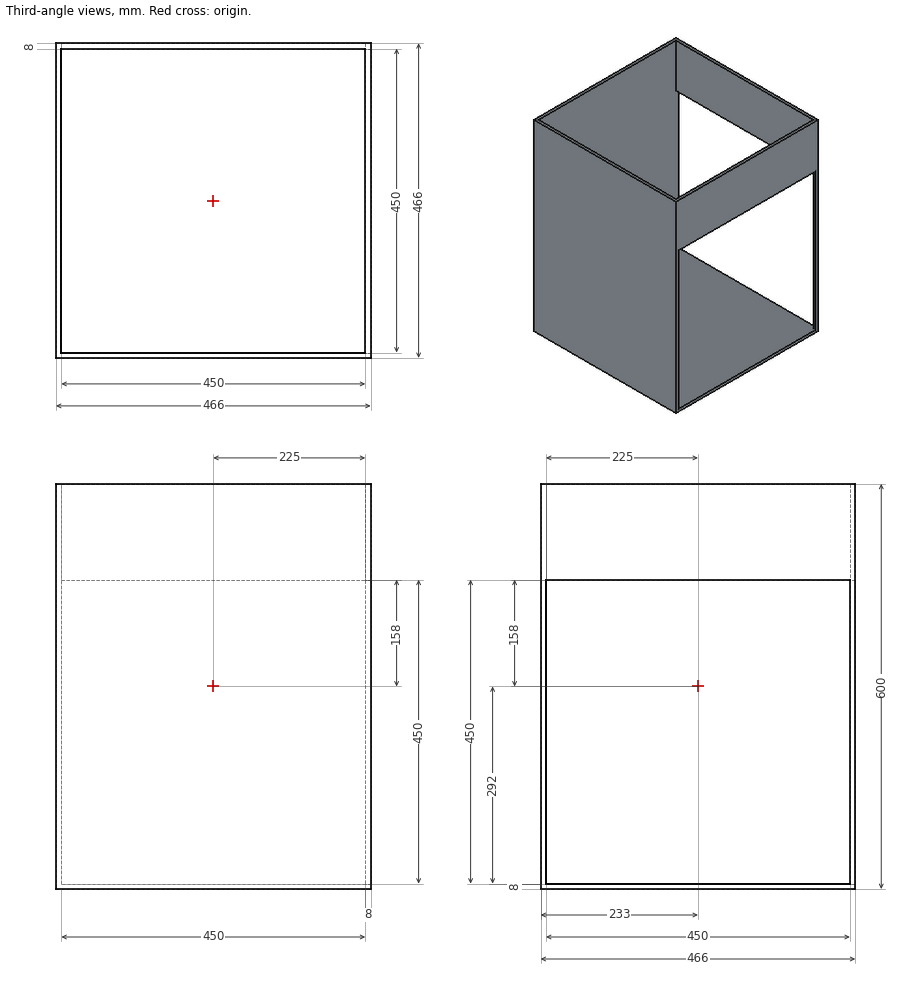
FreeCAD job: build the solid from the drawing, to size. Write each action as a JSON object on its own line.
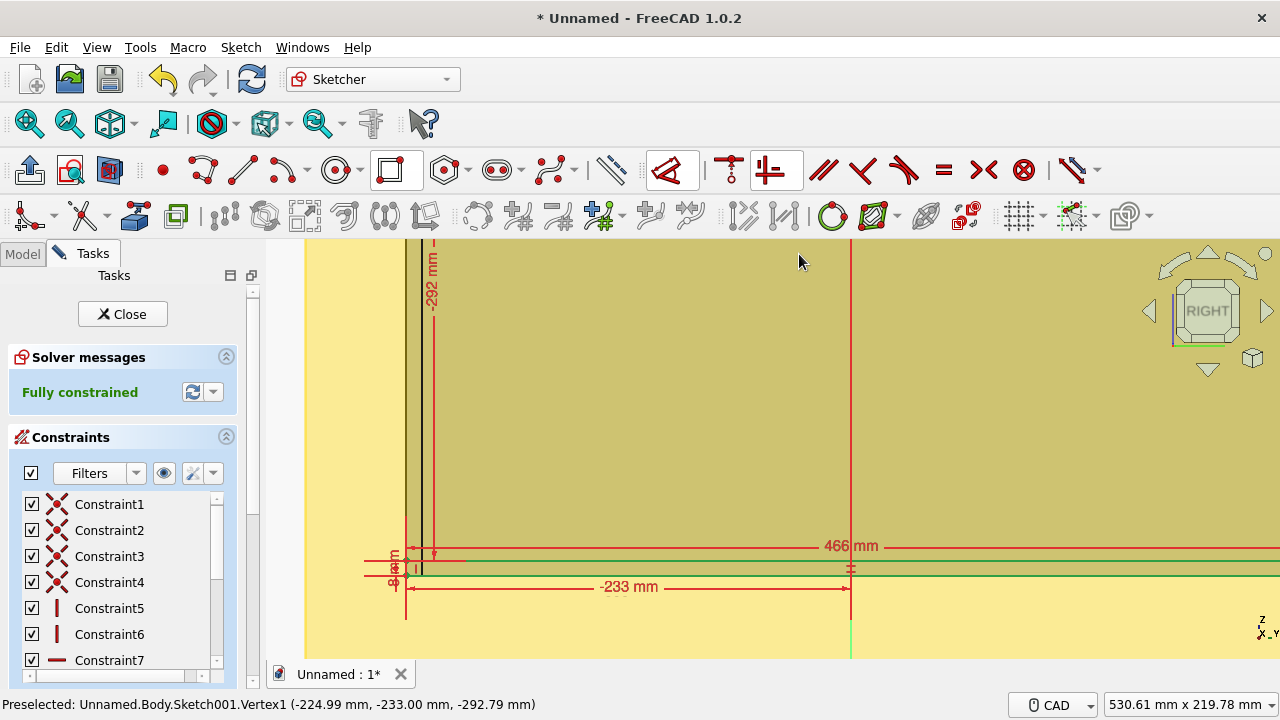
{"action": "left_click", "coordinate": [123, 314]}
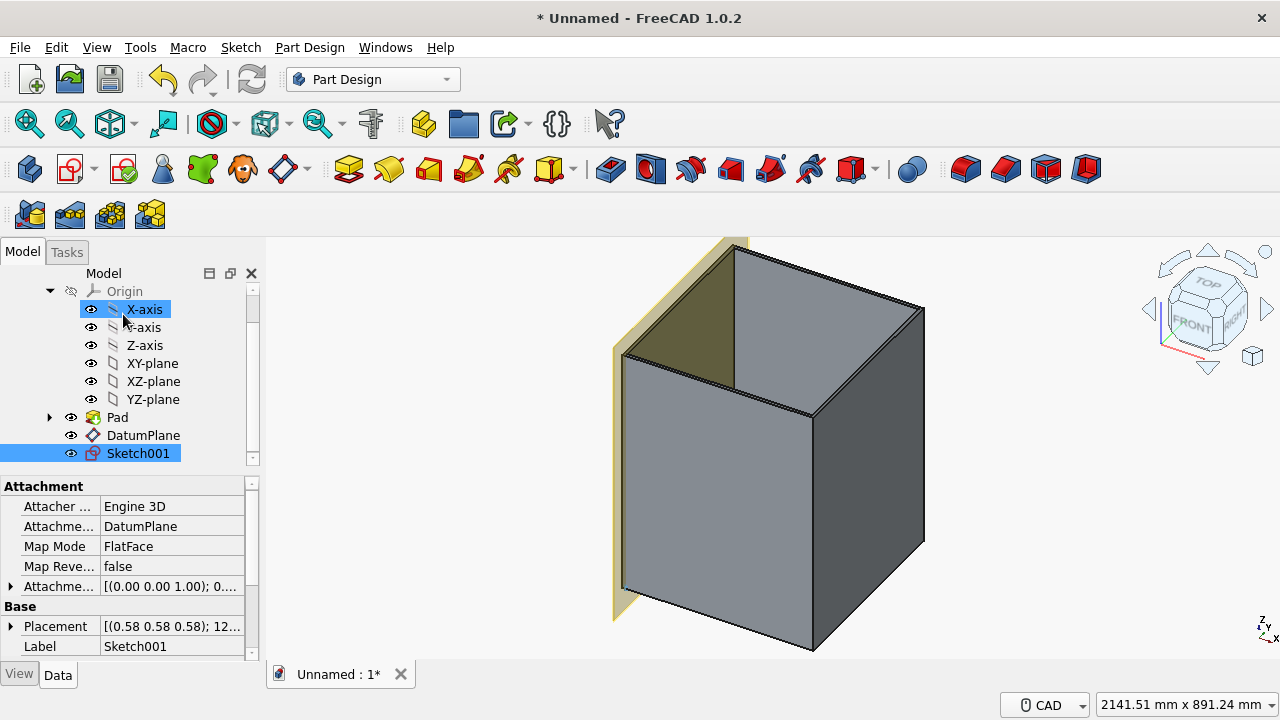
{"action": "left_click", "coordinate": [350, 170]}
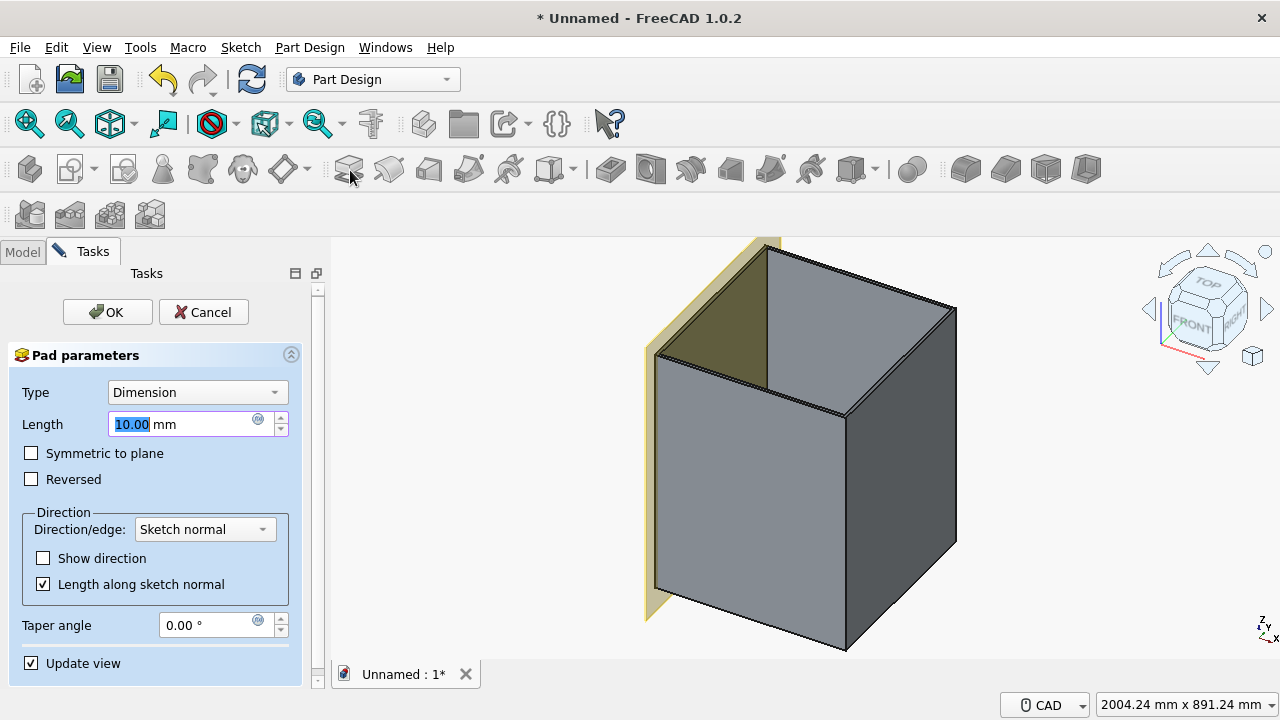
{"action": "type", "text": "450"}
{"action": "key", "text": "Tab"}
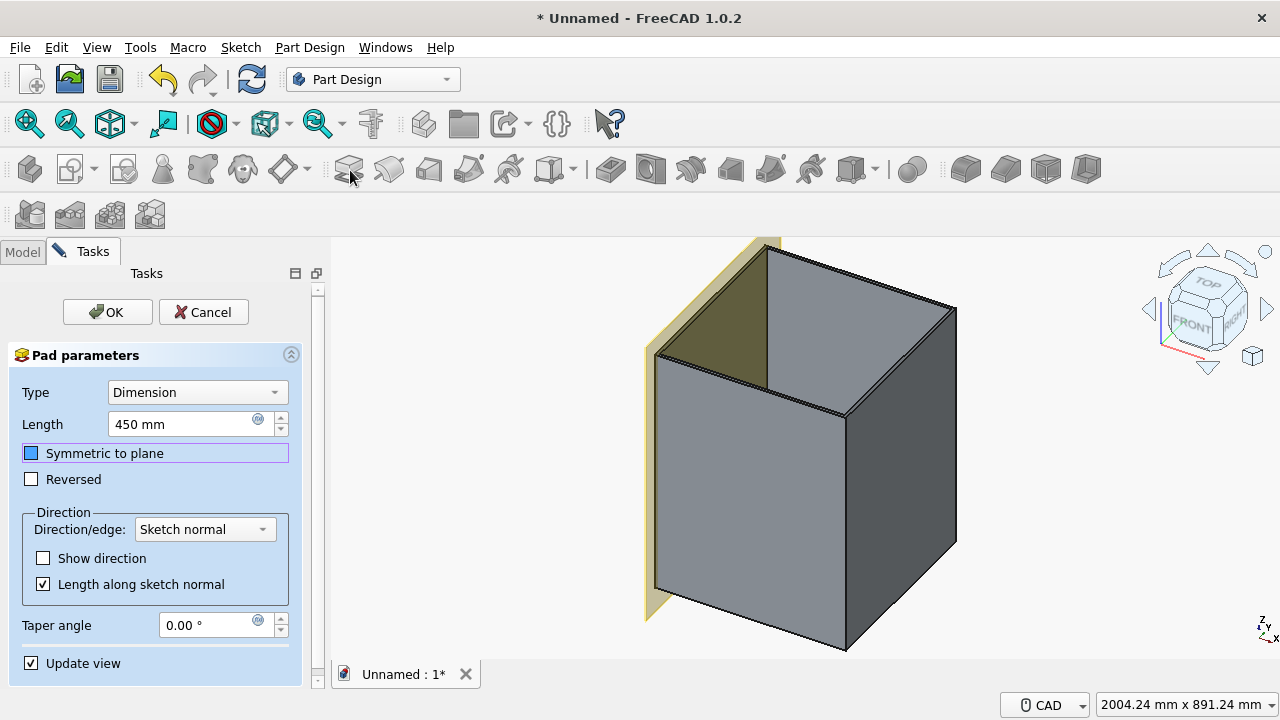
{"action": "left_click", "coordinate": [108, 312]}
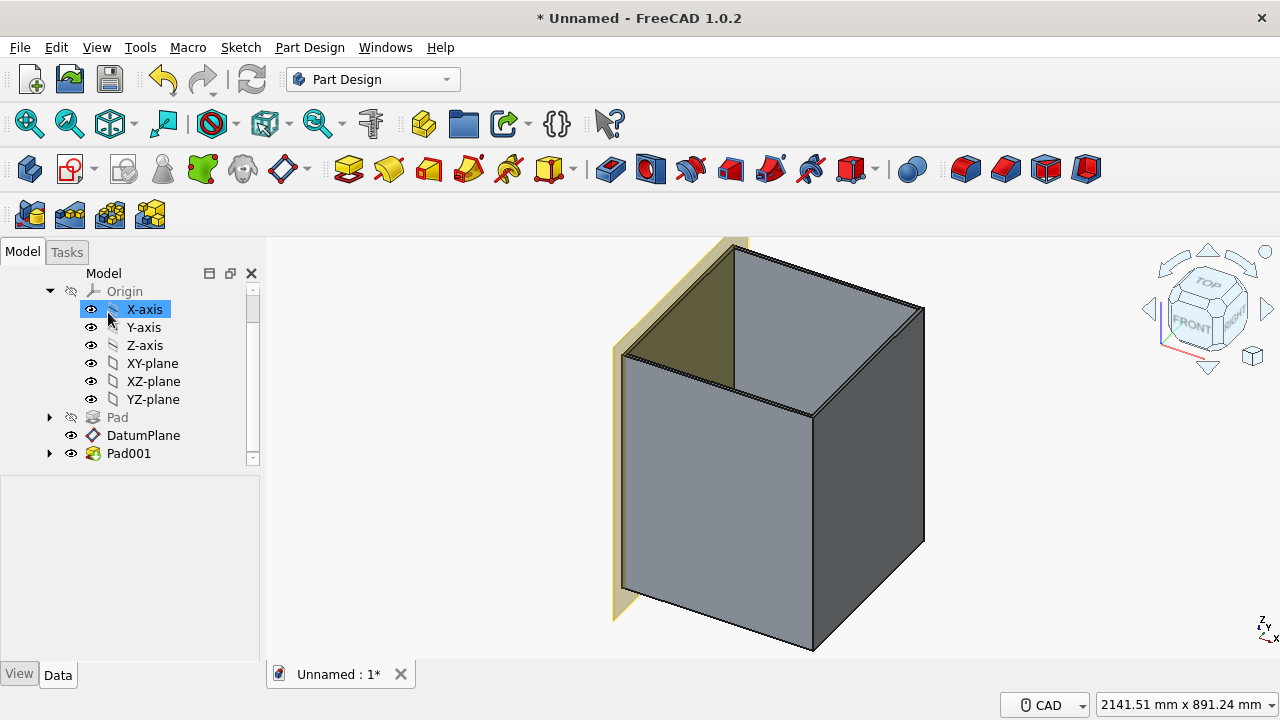
{"action": "left_click", "coordinate": [116, 435]}
{"action": "key", "text": "space"}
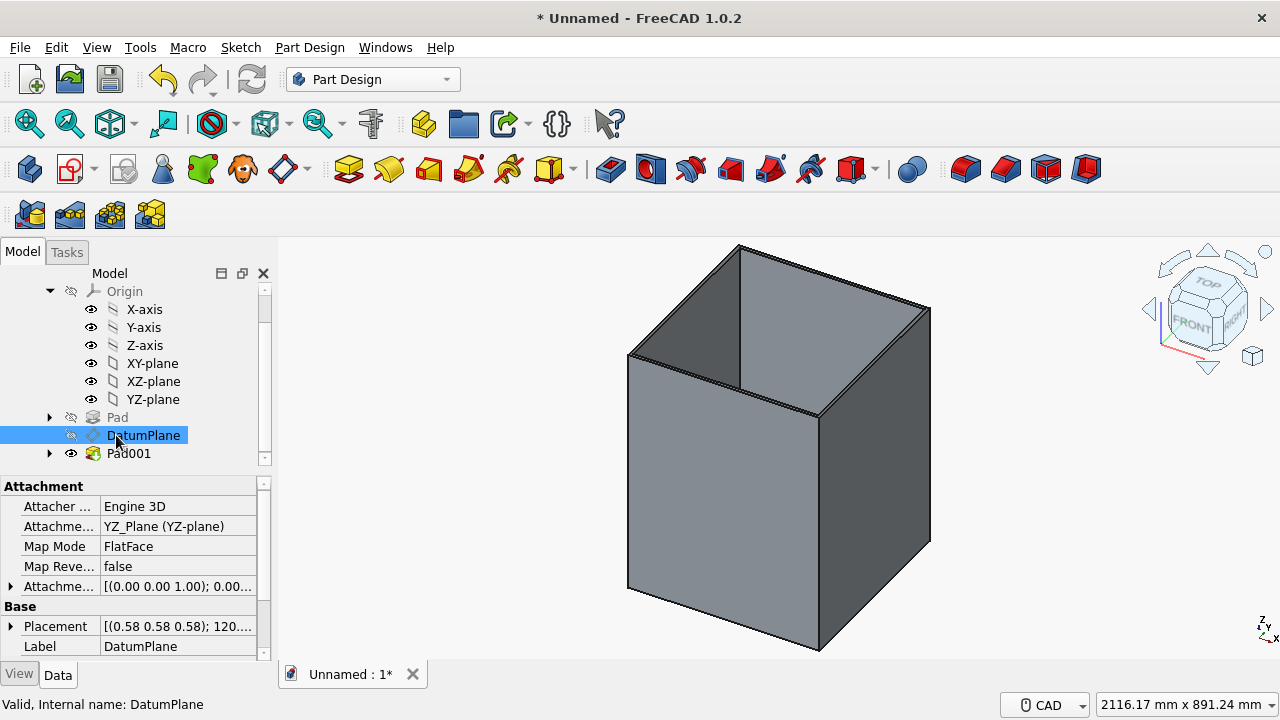
{"action": "key", "text": "4"}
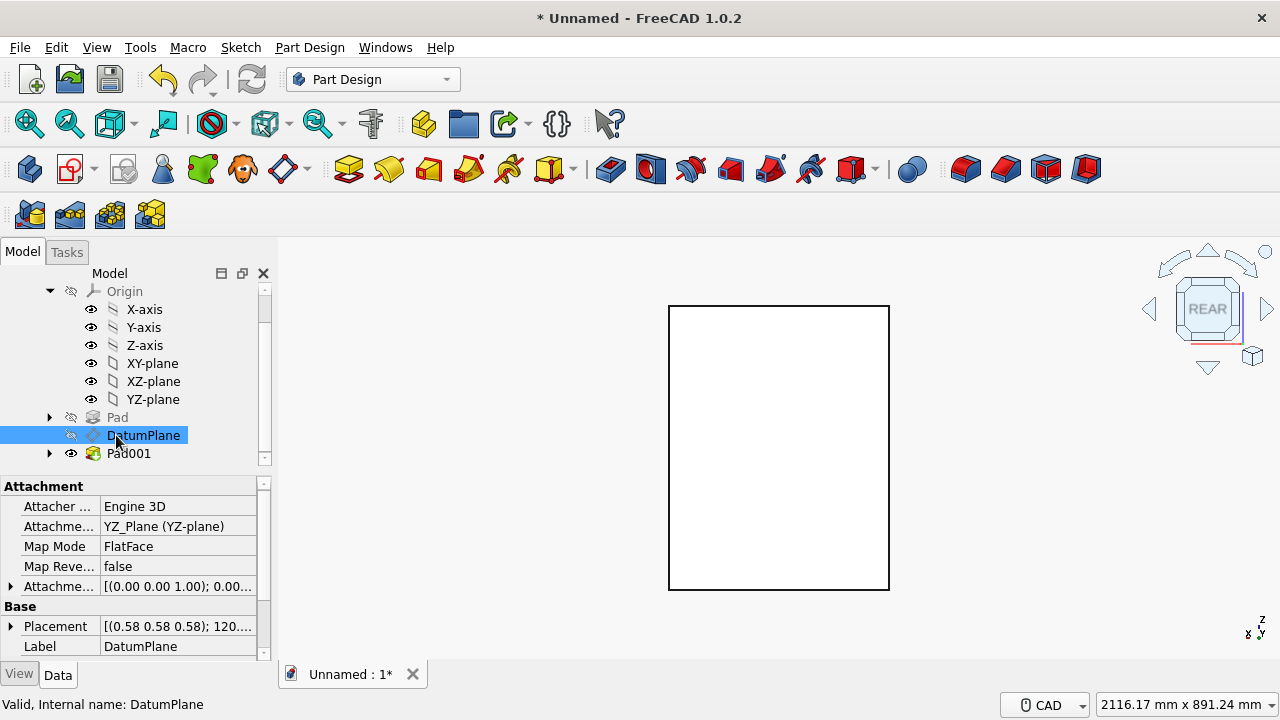
{"action": "left_click", "coordinate": [779, 447]}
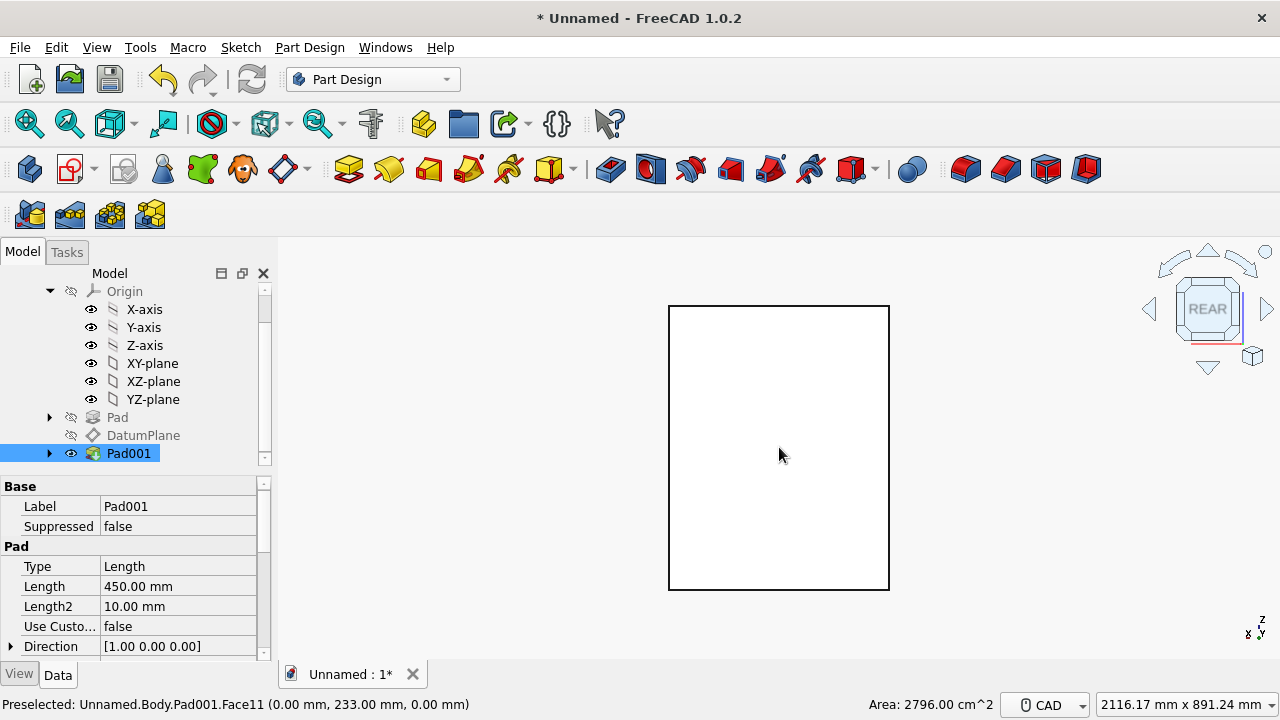
{"action": "left_click", "coordinate": [70, 170]}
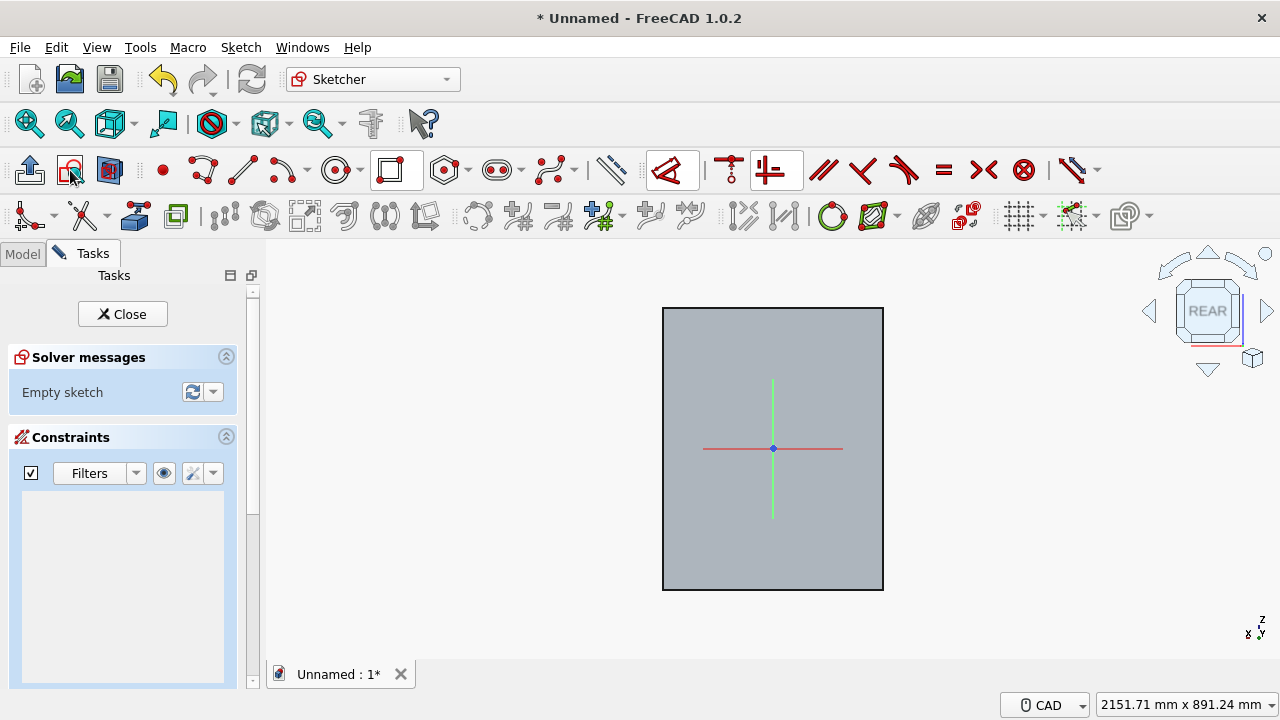
{"action": "left_click", "coordinate": [390, 170]}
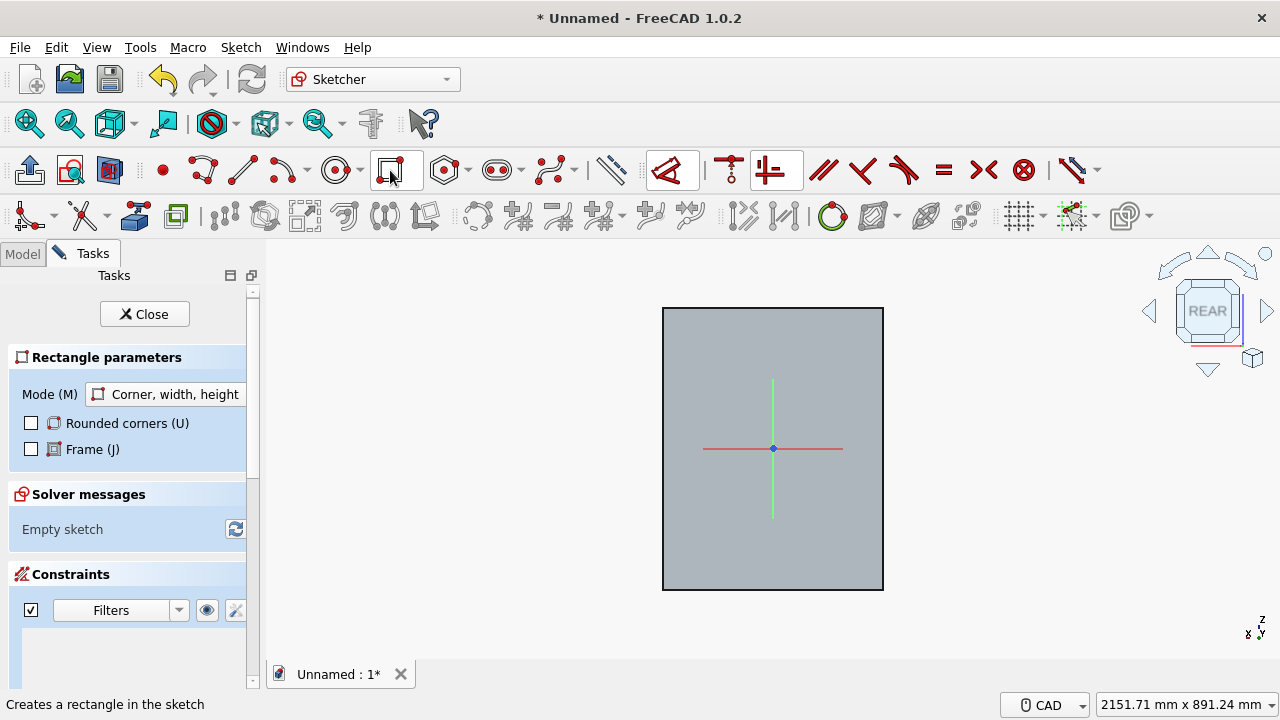
{"action": "left_click", "coordinate": [667, 375]}
{"action": "left_click", "coordinate": [879, 587]}
{"action": "key", "text": "Escape"}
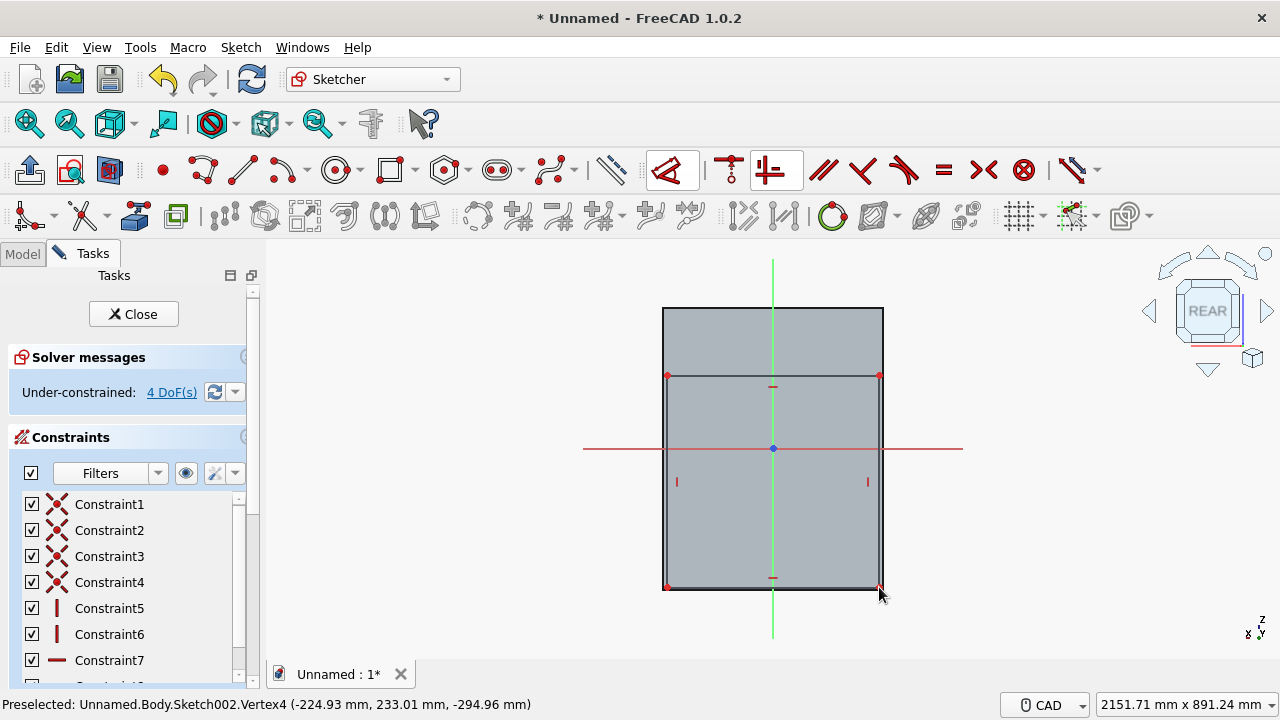
{"action": "scroll", "coordinate": [667, 440], "scroll_direction": "up", "scroll_amount": 2}